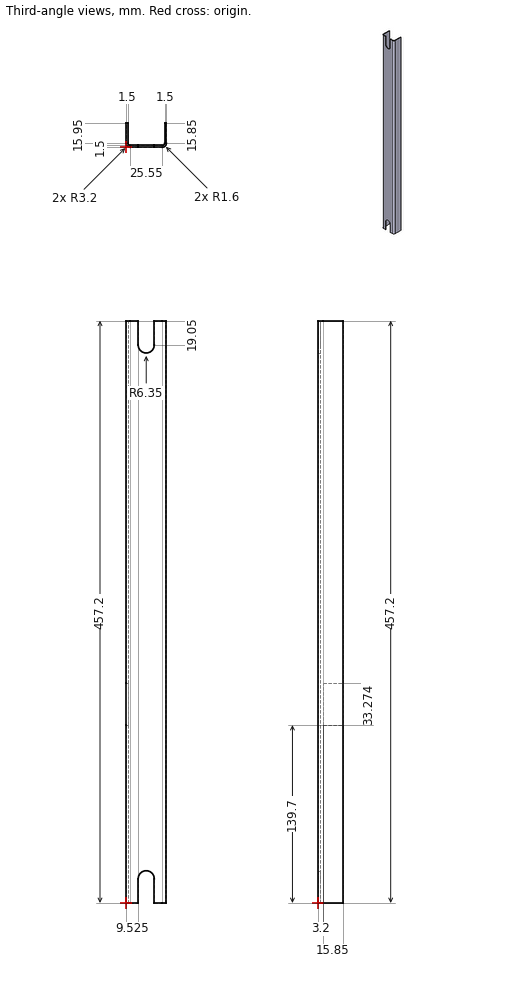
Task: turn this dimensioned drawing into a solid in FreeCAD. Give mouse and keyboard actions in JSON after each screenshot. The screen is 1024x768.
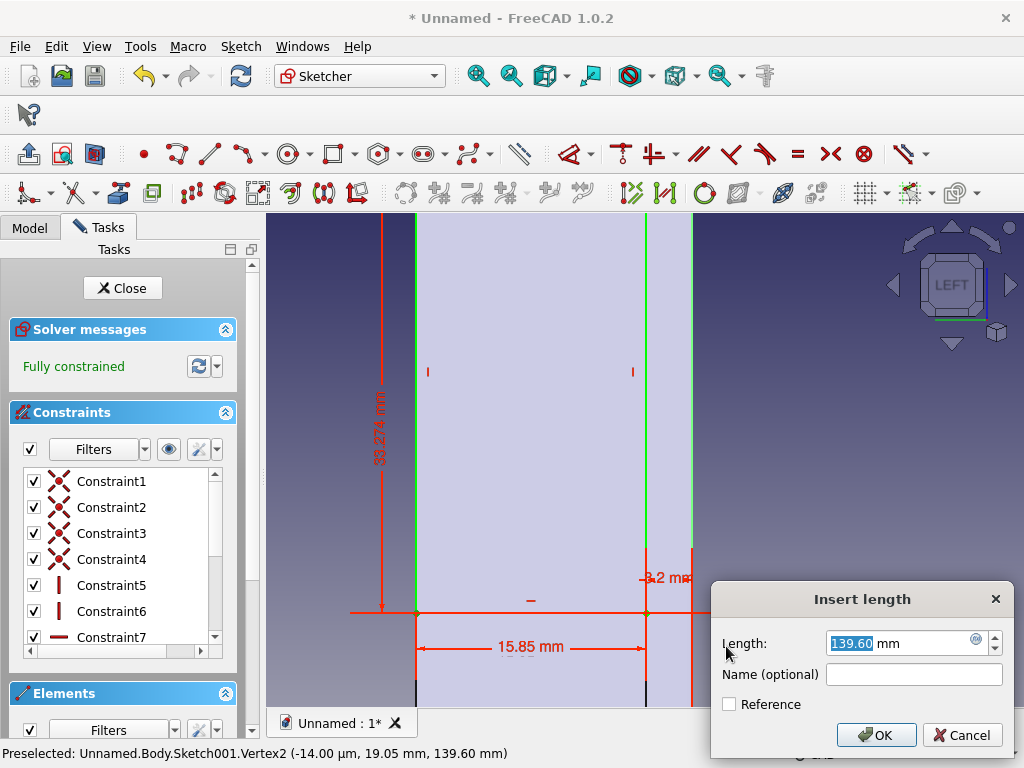
{"action": "type", "text": "139.7"}
{"action": "key", "text": "Return"}
{"action": "key", "text": "Escape"}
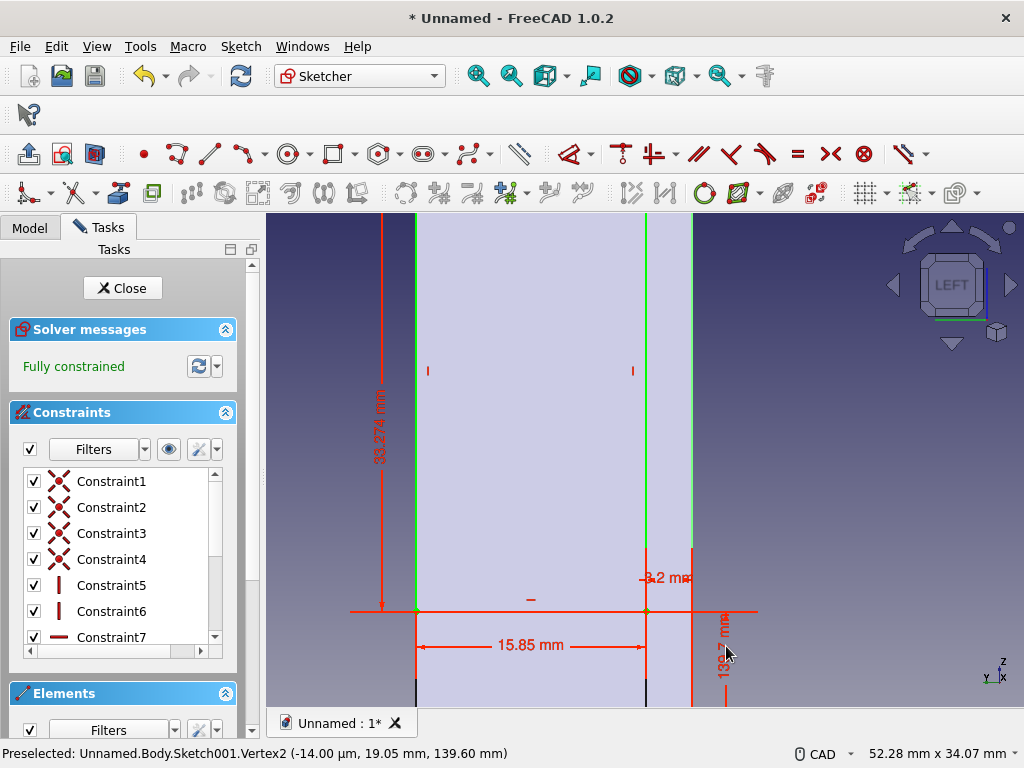
{"action": "left_click", "coordinate": [123, 288]}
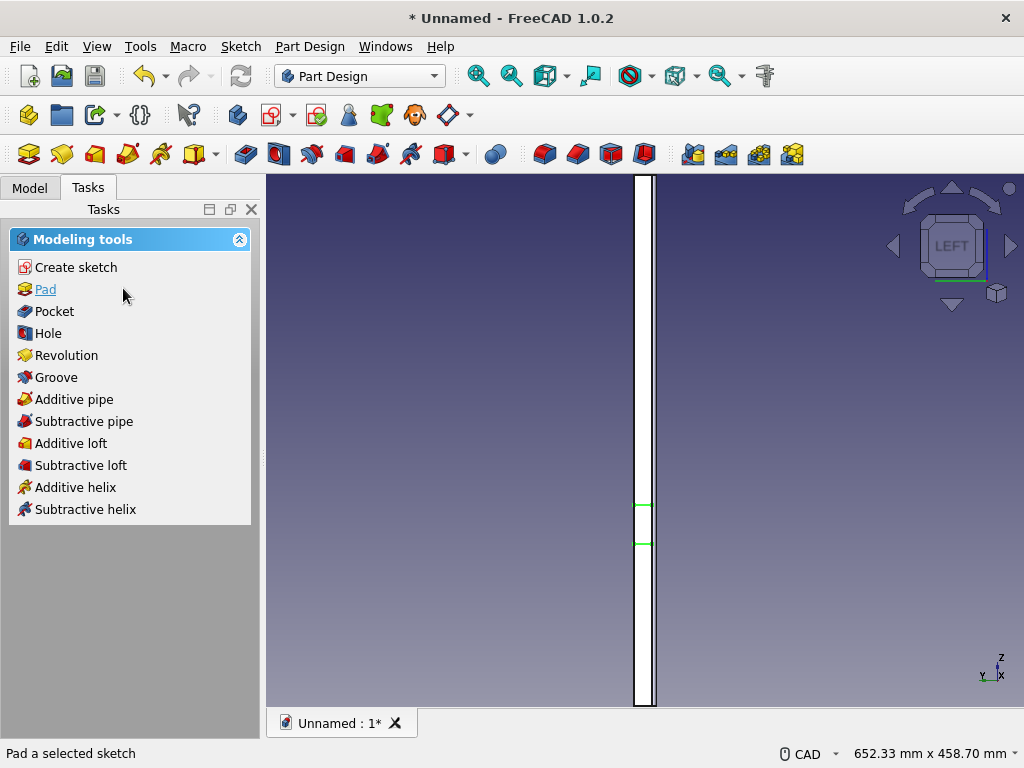
{"action": "left_click", "coordinate": [246, 154]}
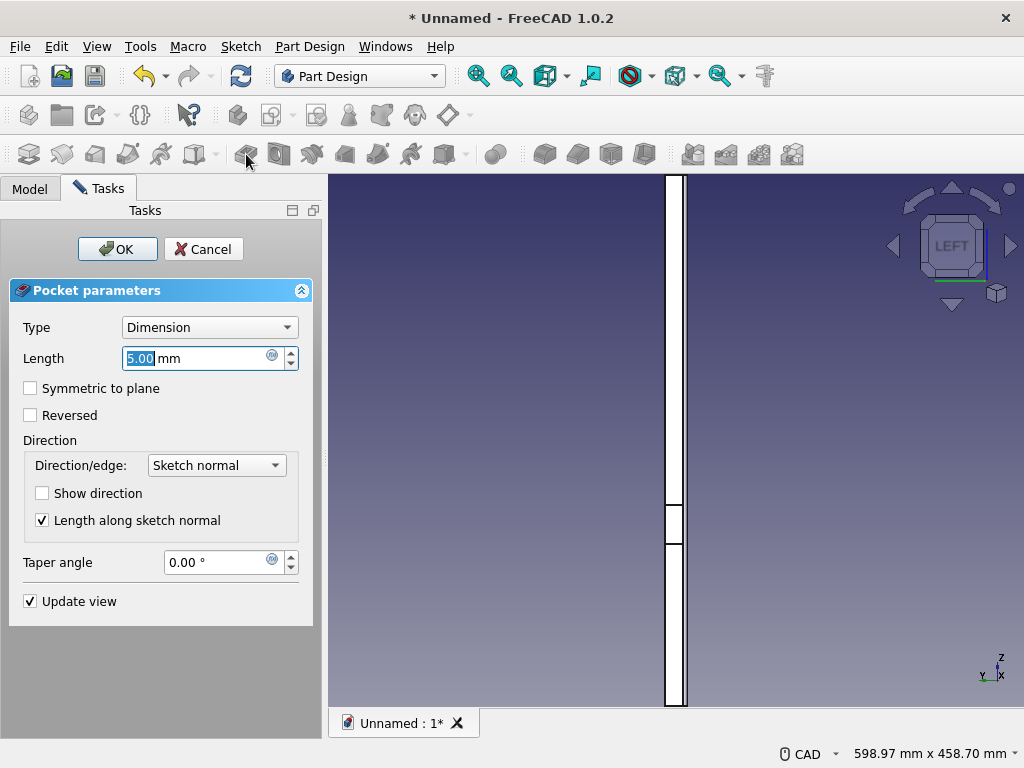
{"action": "left_click", "coordinate": [210, 328]}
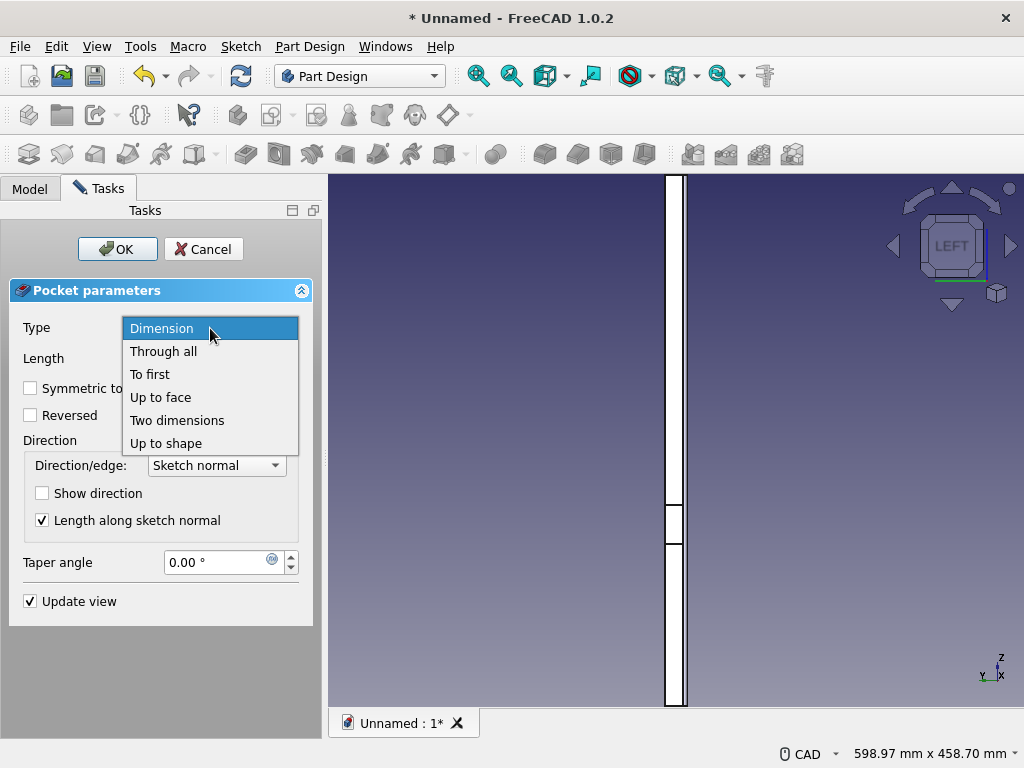
{"action": "left_click", "coordinate": [208, 374]}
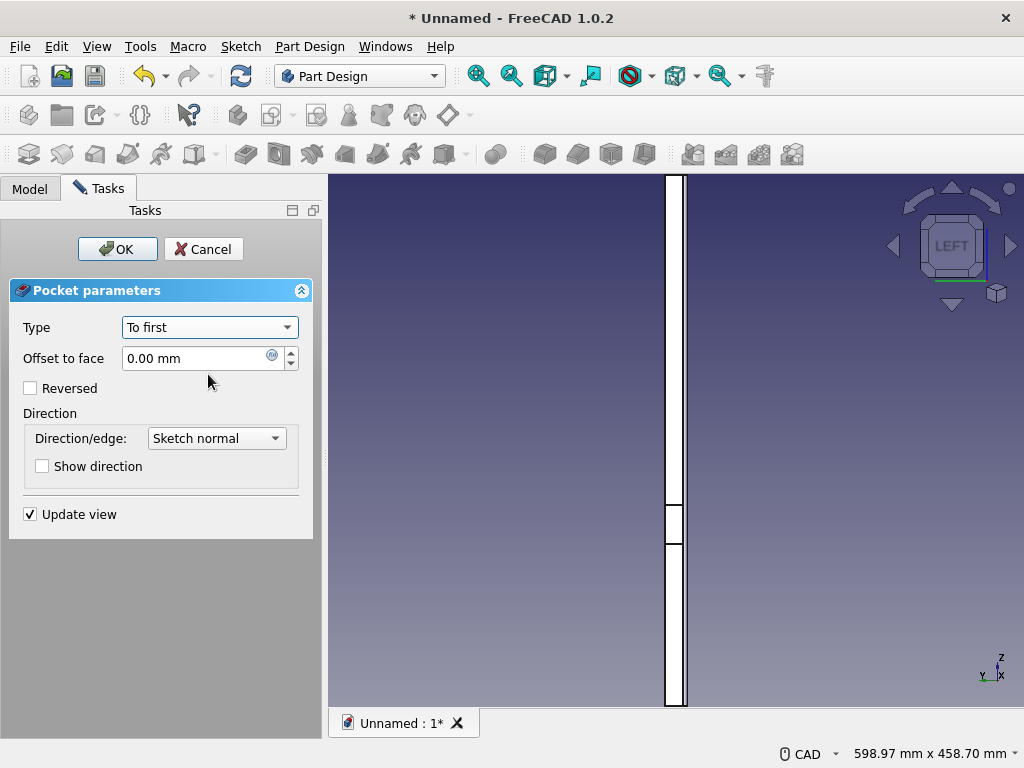
{"action": "left_click", "coordinate": [118, 249]}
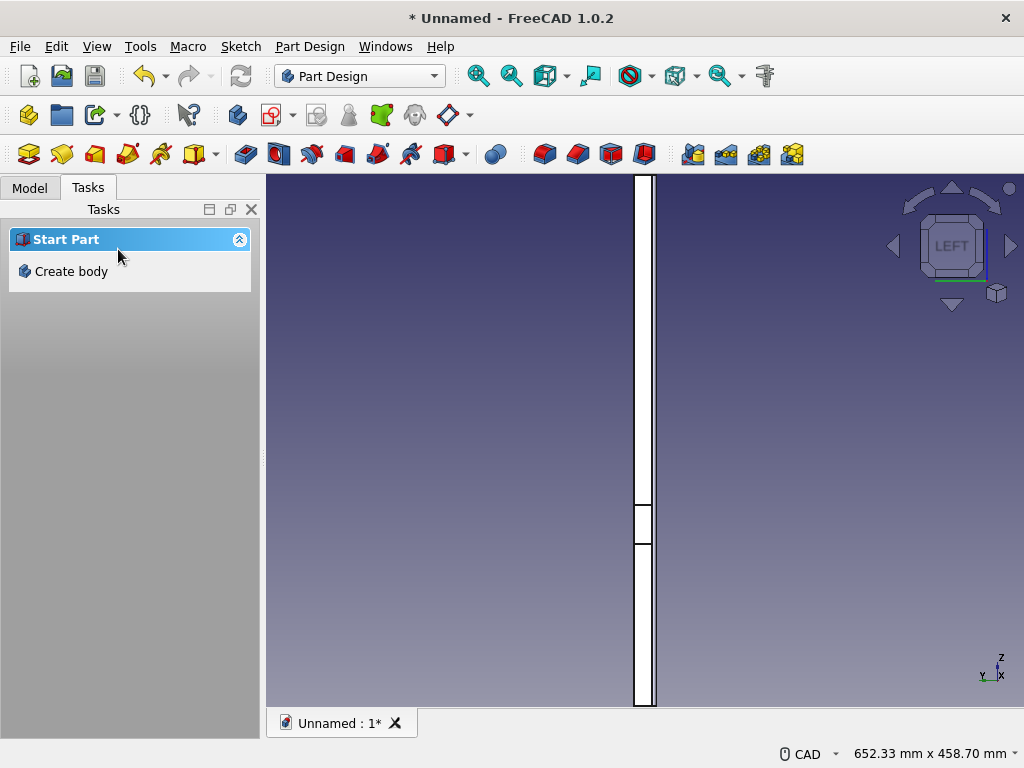
{"action": "key", "text": "0"}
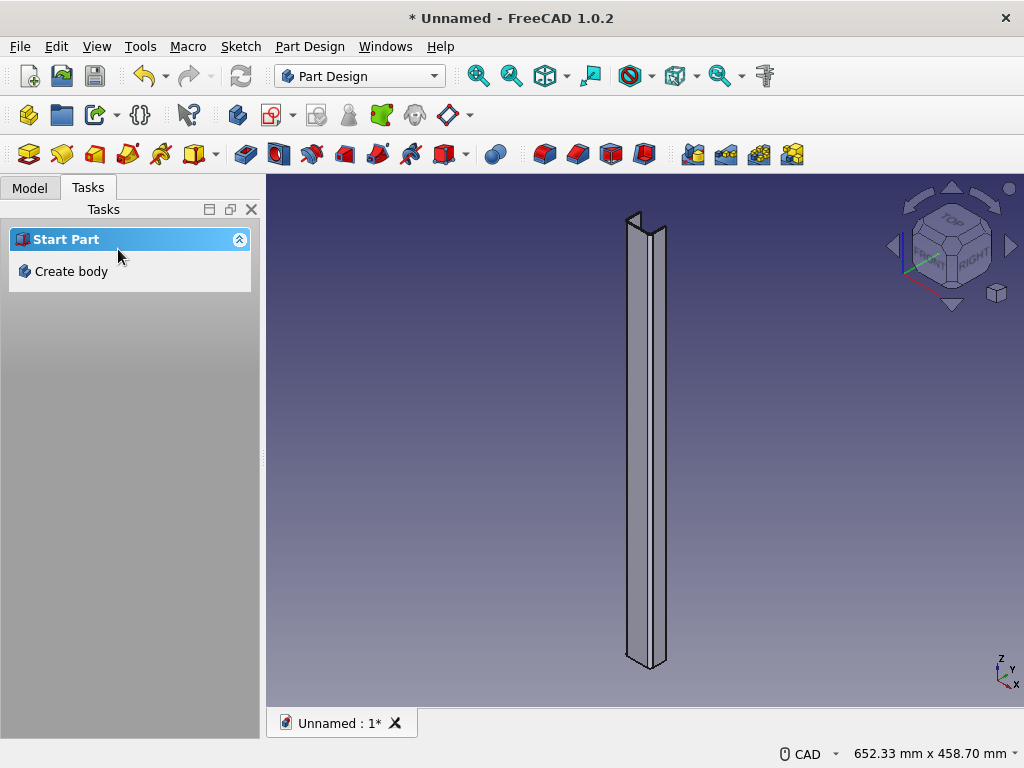
{"action": "left_click", "coordinate": [637, 258]}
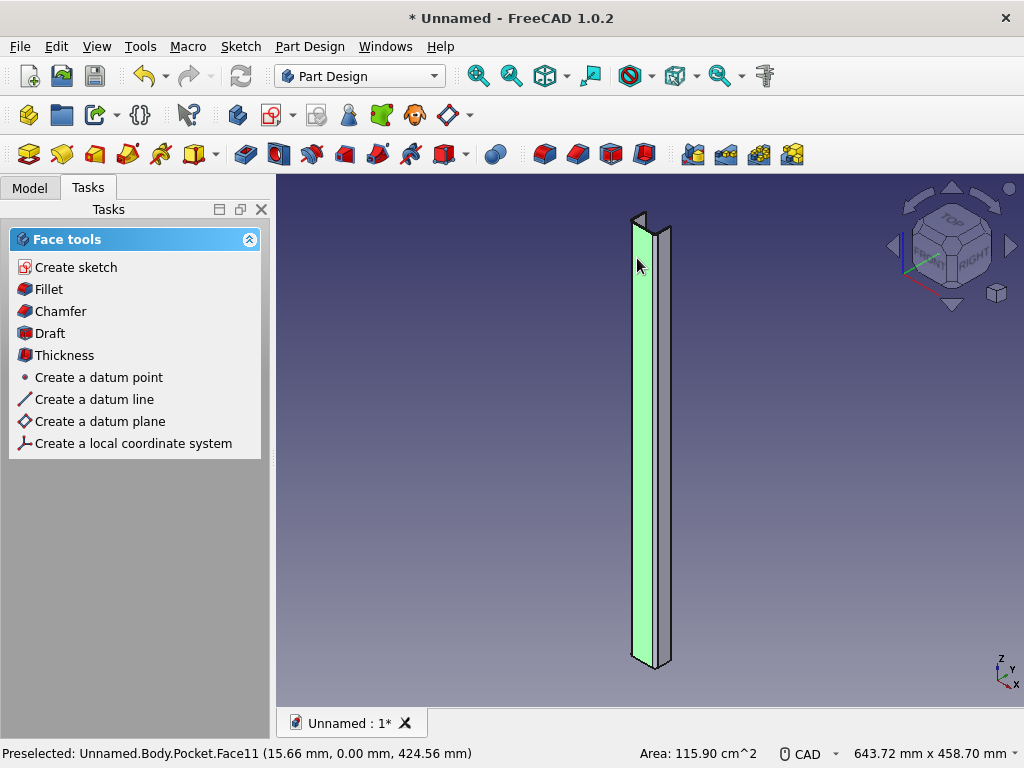
{"action": "left_click", "coordinate": [270, 116]}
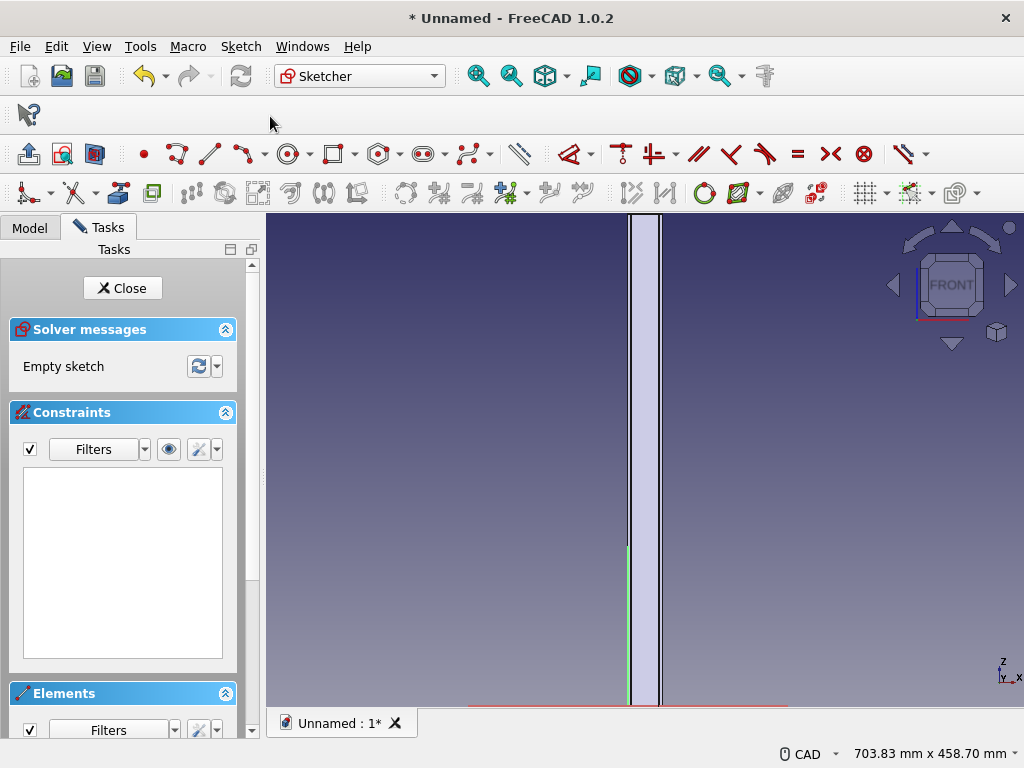
{"action": "scroll", "coordinate": [576, 460], "scroll_direction": "down", "scroll_amount": 5}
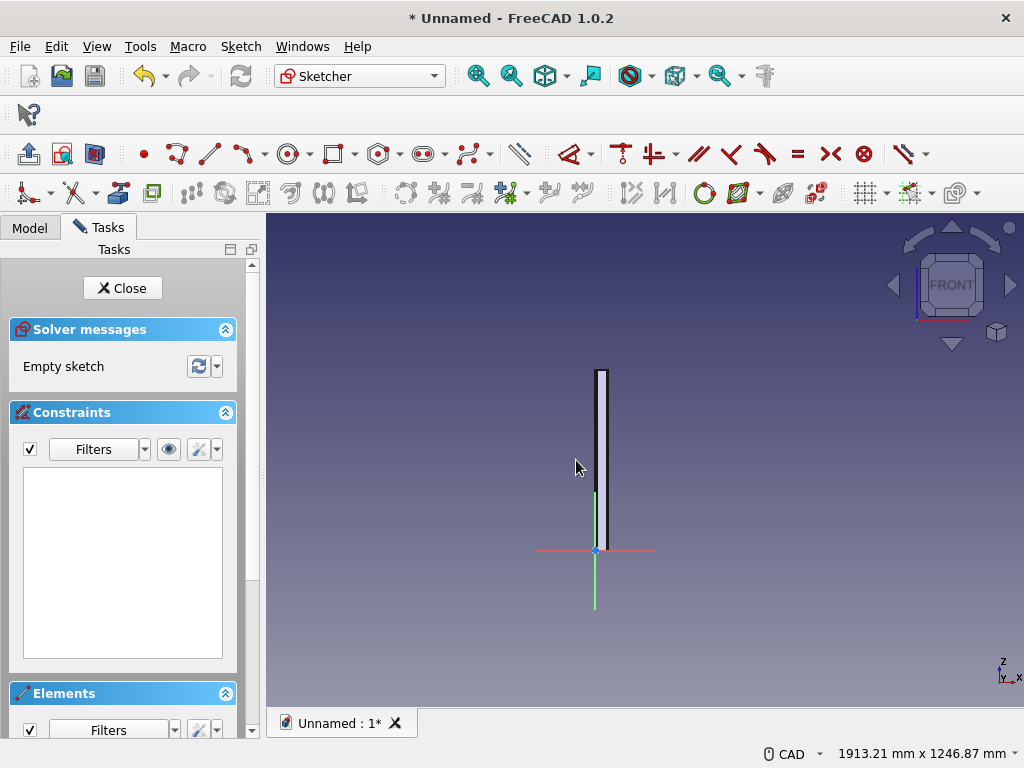
{"action": "scroll", "coordinate": [603, 370], "scroll_direction": "up", "scroll_amount": 15}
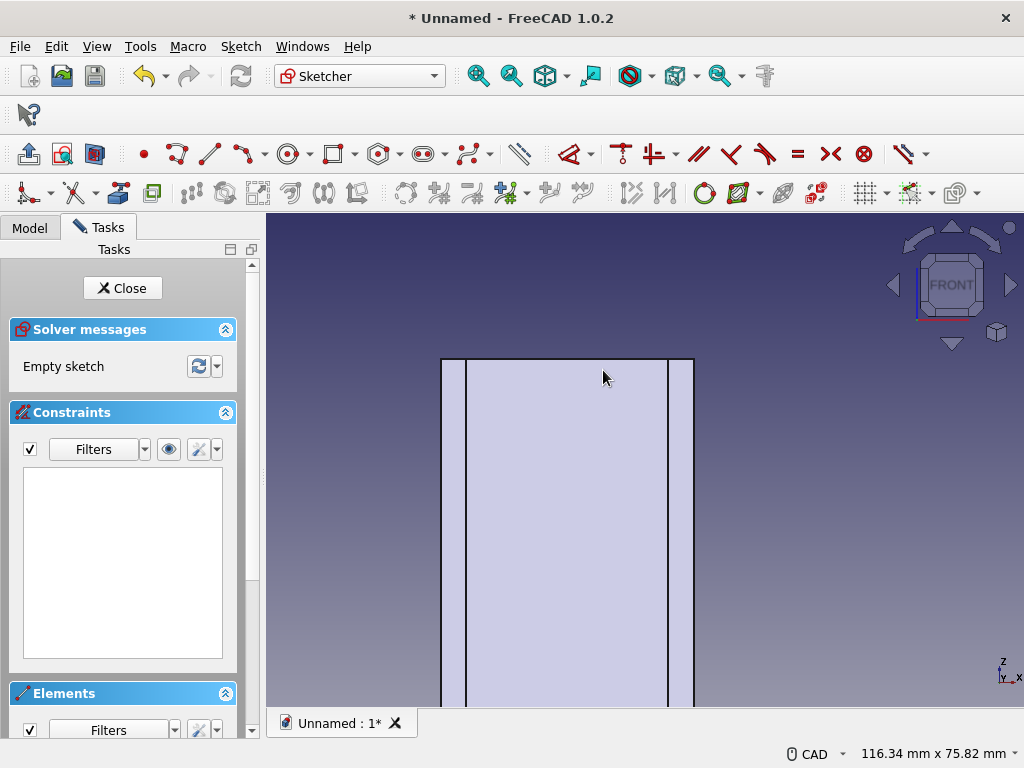
{"action": "scroll", "coordinate": [548, 460], "scroll_direction": "up", "scroll_amount": 2}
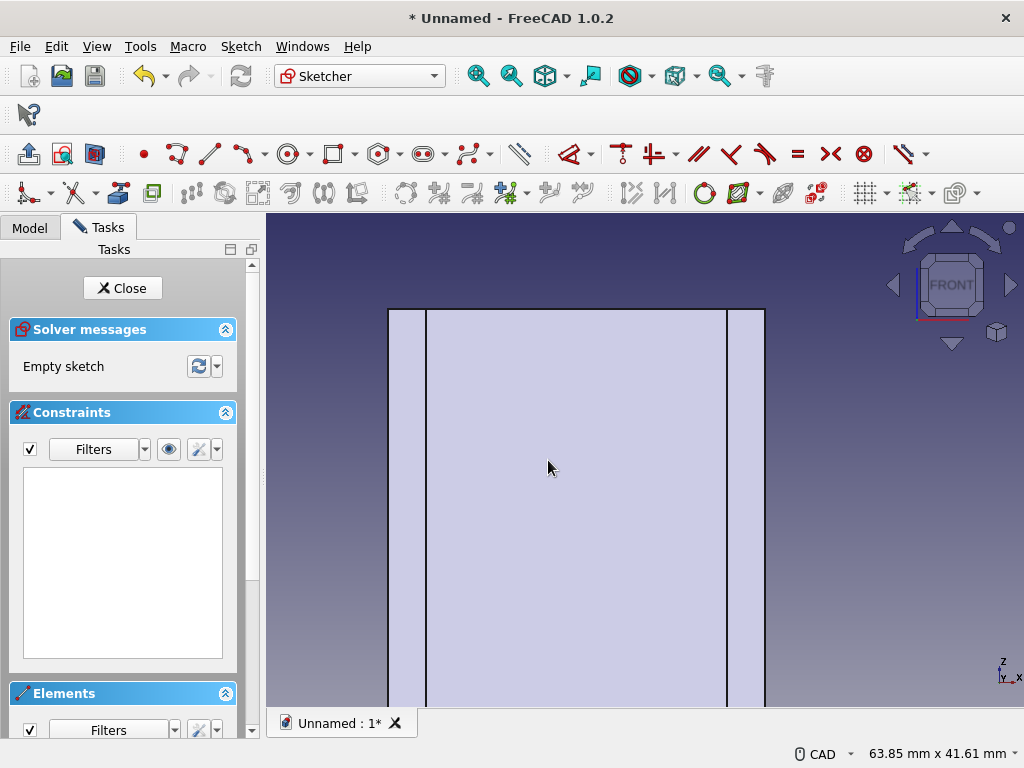
{"action": "left_click", "coordinate": [177, 154]}